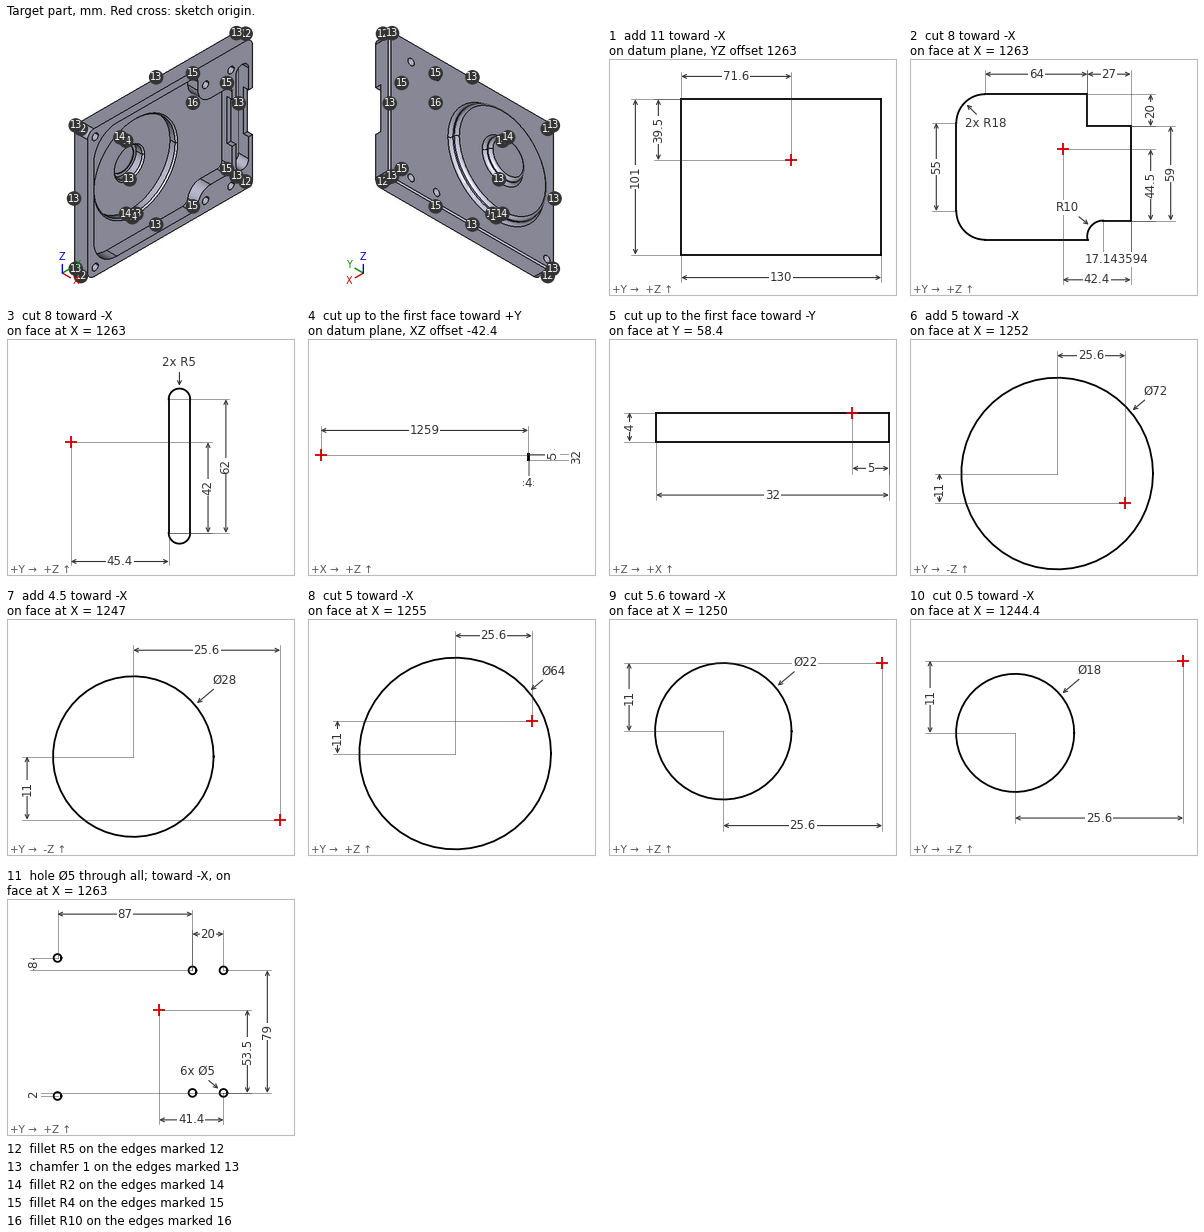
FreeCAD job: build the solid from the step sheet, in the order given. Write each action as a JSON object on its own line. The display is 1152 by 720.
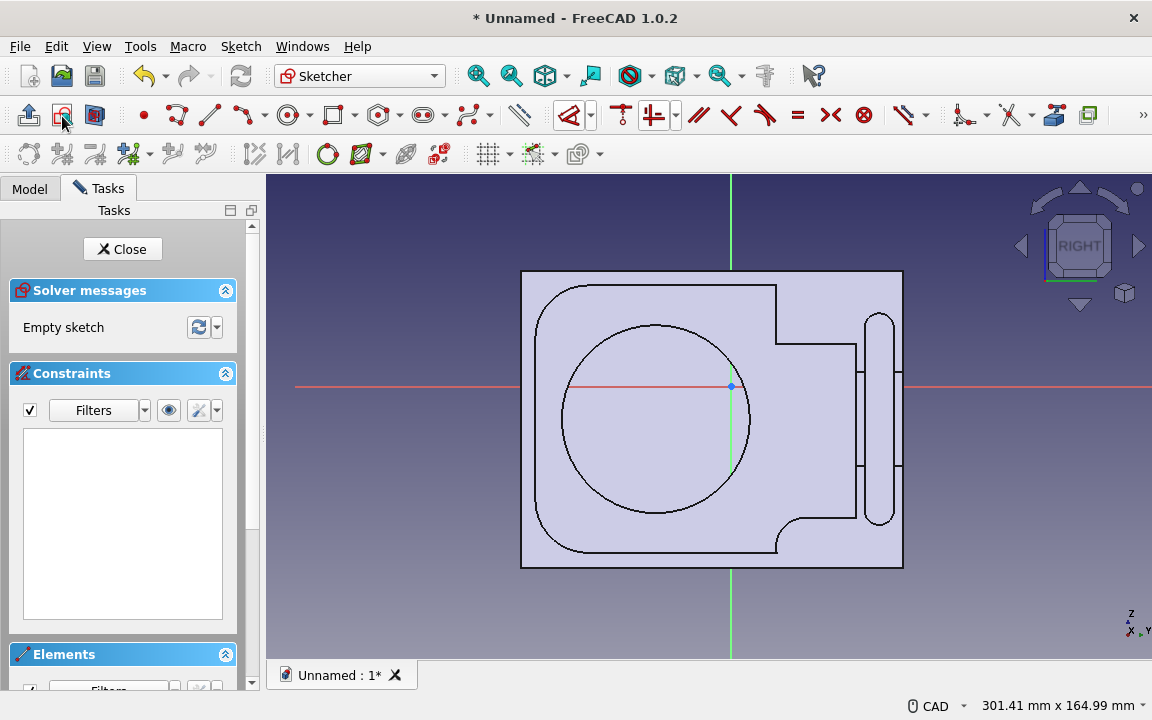
{"action": "left_click", "coordinate": [95, 116]}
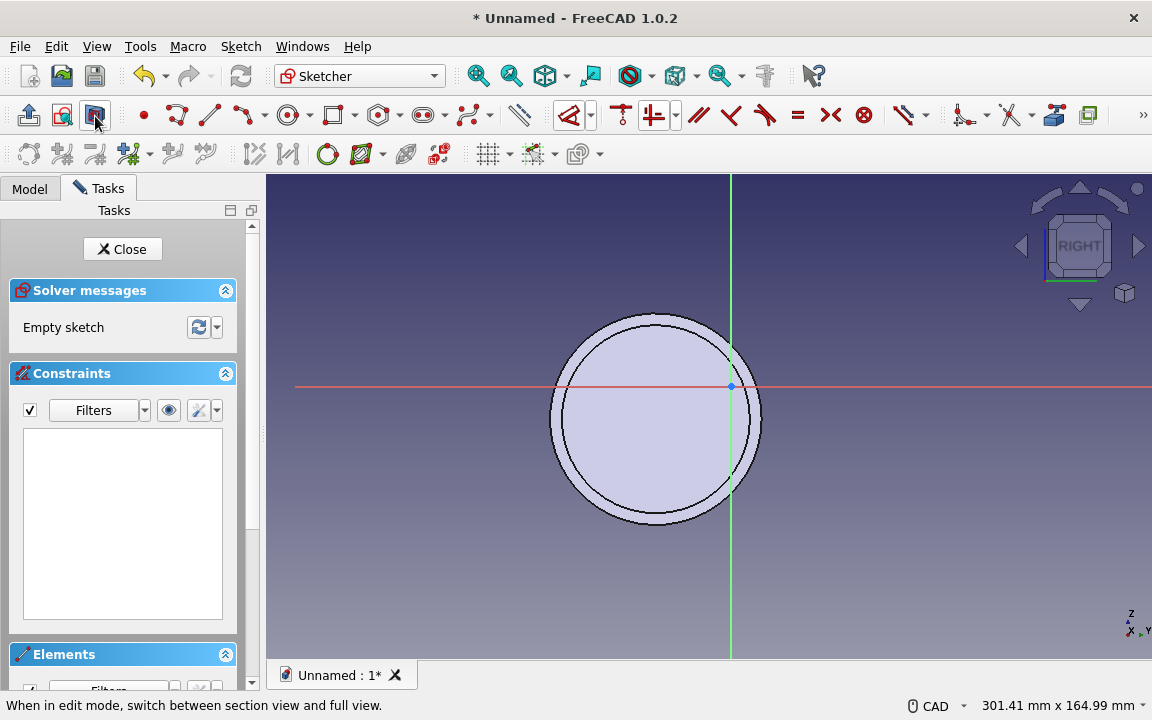
{"action": "scroll", "coordinate": [687, 420], "scroll_direction": "up", "scroll_amount": 8}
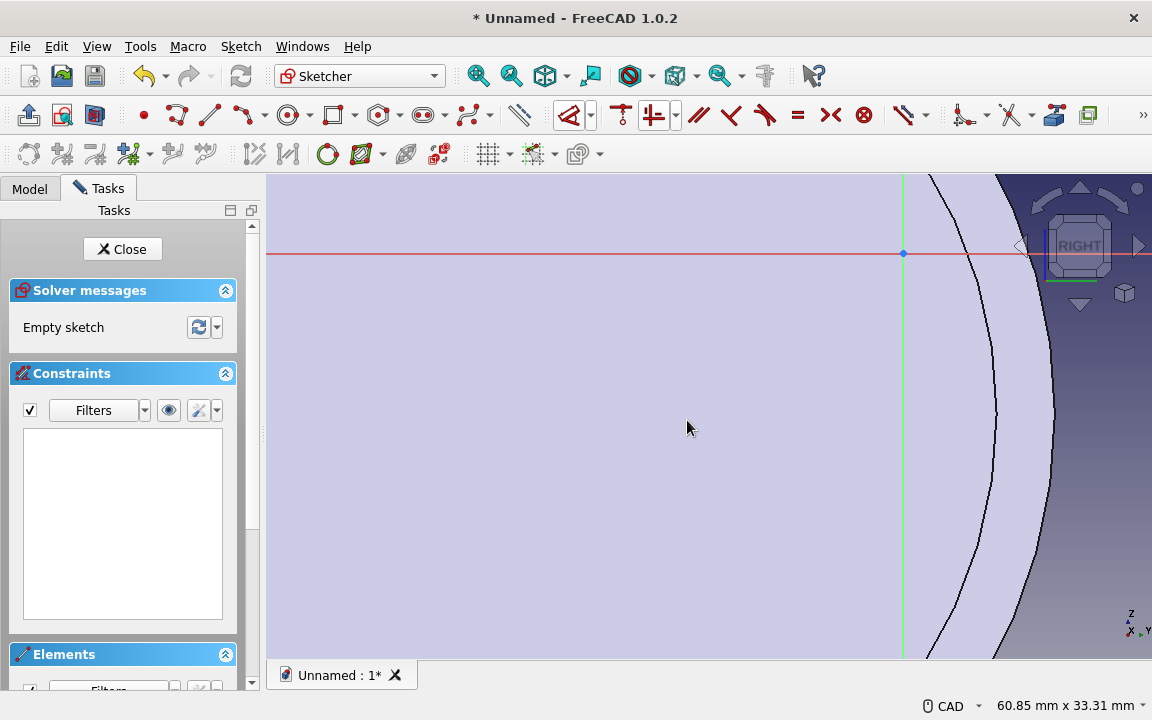
{"action": "left_click", "coordinate": [288, 116]}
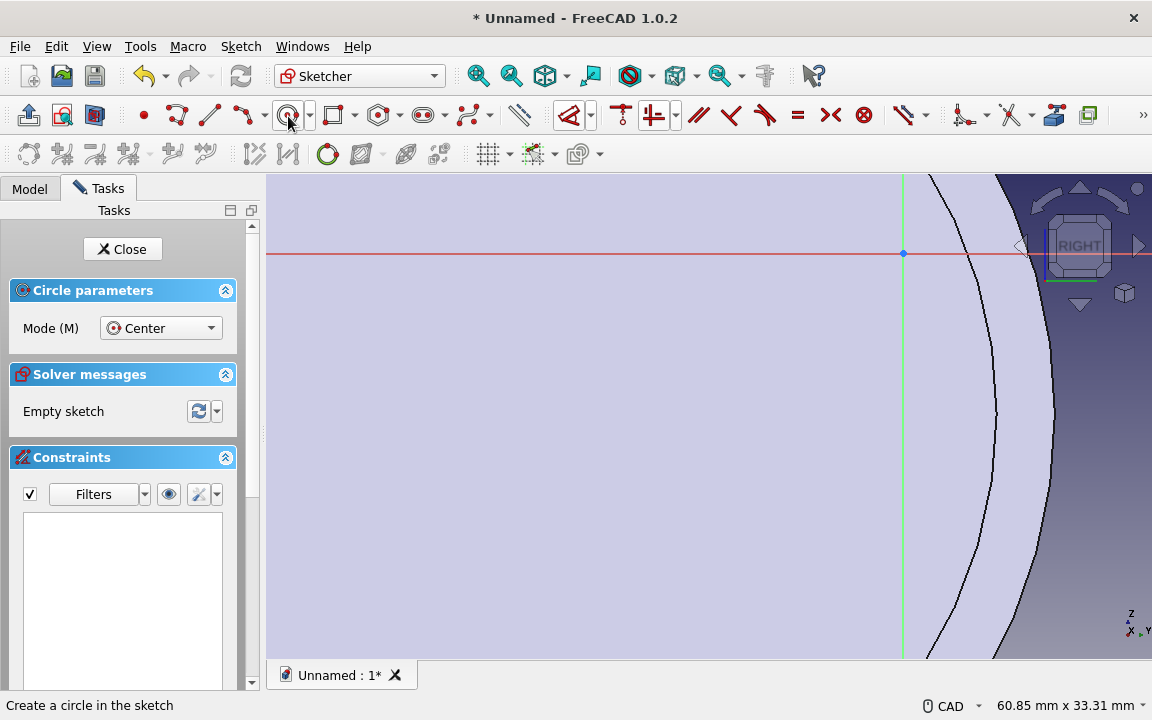
{"action": "left_click", "coordinate": [531, 414]}
{"action": "left_click", "coordinate": [644, 301]}
{"action": "key", "text": "Escape"}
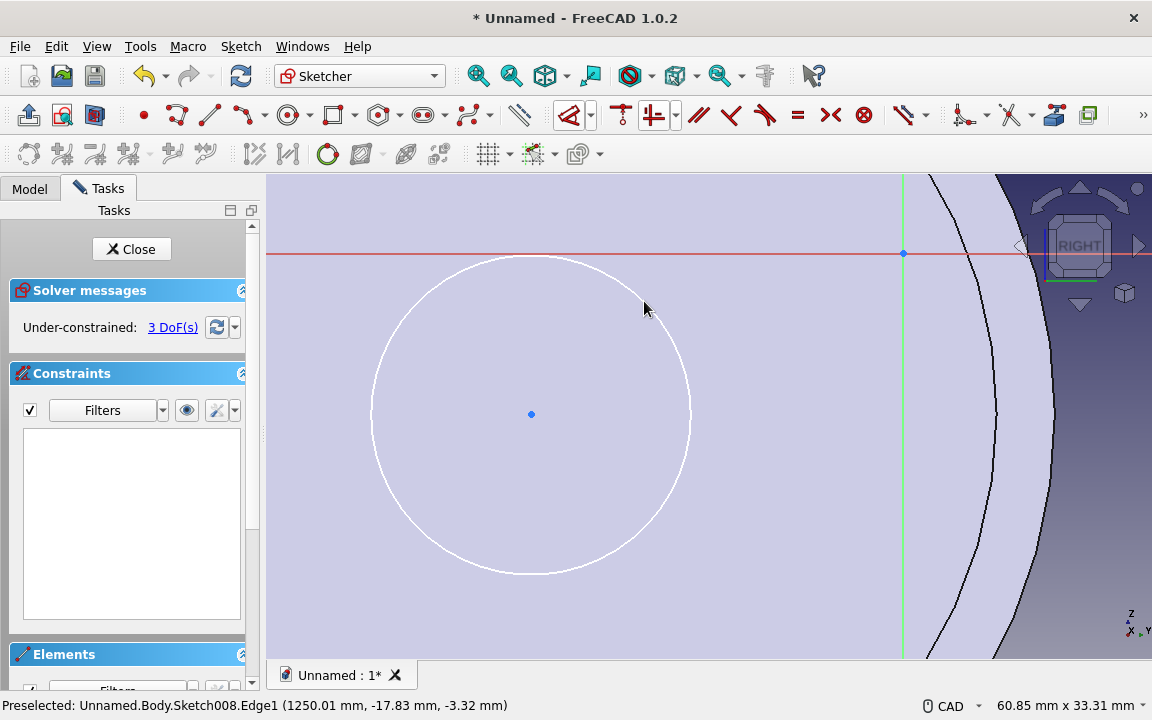
{"action": "left_click", "coordinate": [644, 302]}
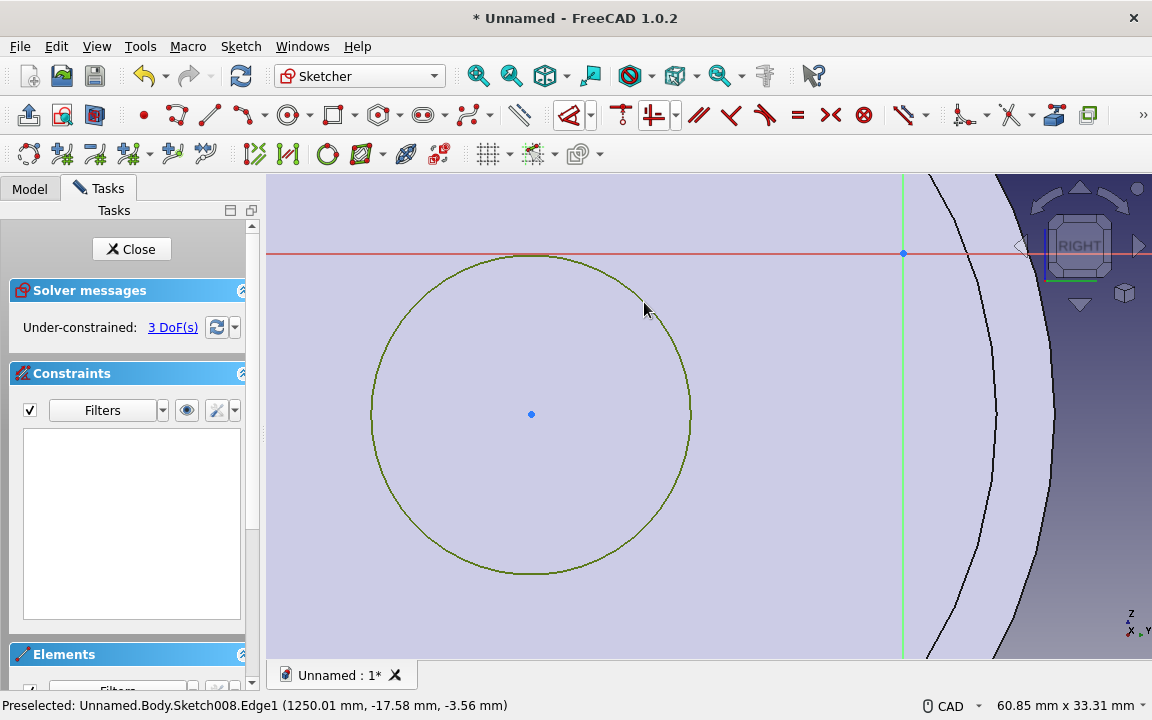
{"action": "key", "text": "k o"}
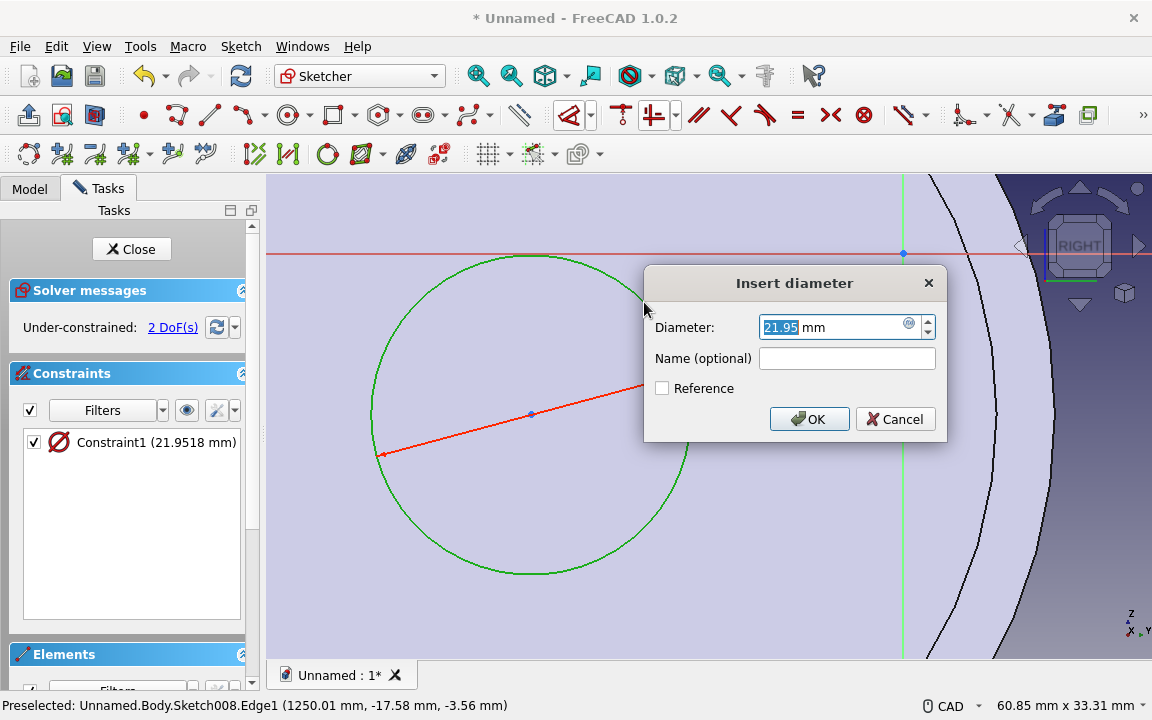
{"action": "type", "text": "22"}
{"action": "key", "text": "Return"}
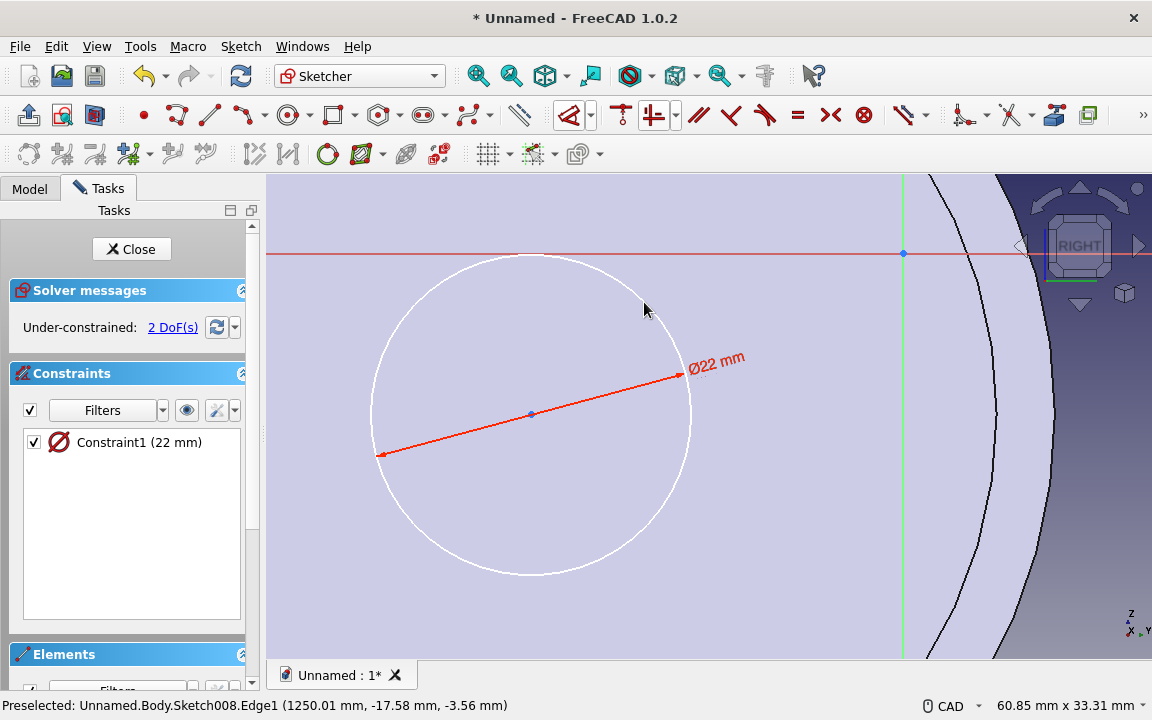
{"action": "left_click", "coordinate": [531, 415]}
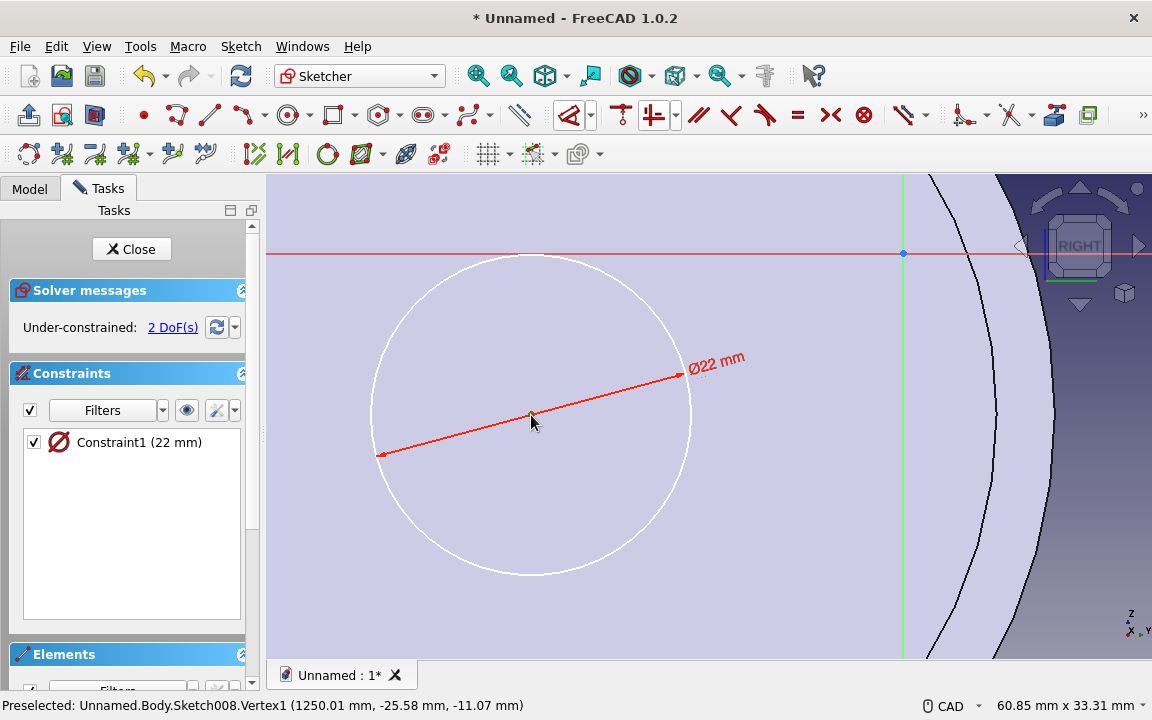
{"action": "key", "text": "i"}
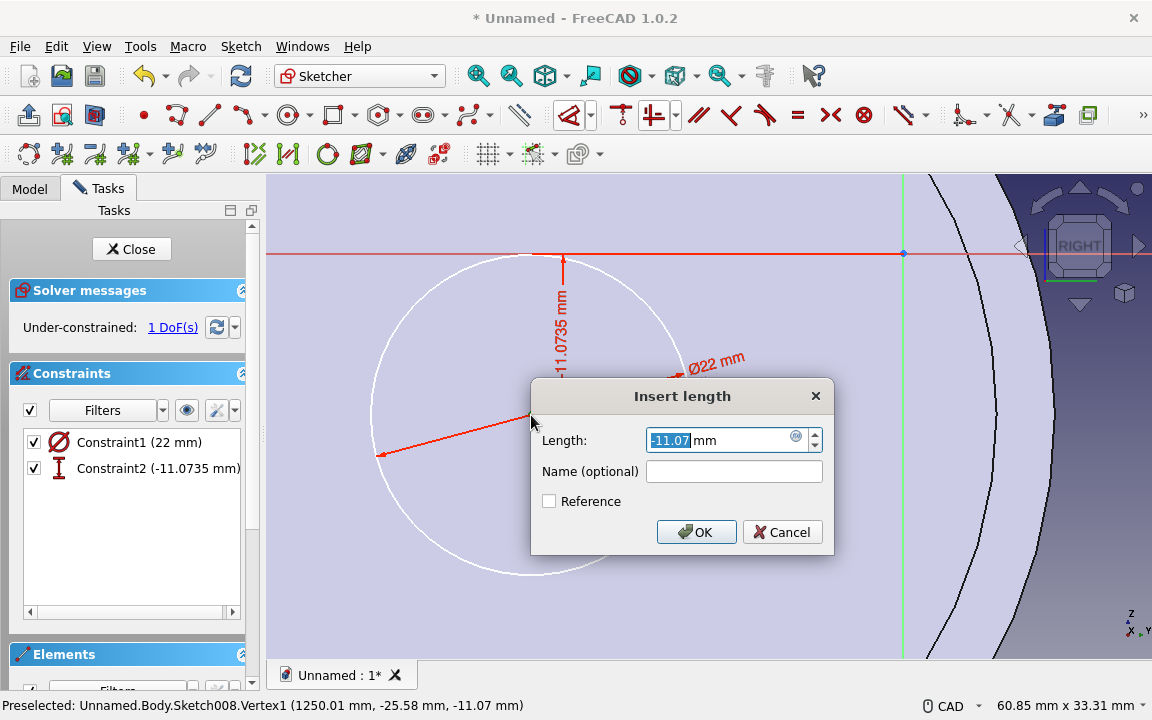
{"action": "type", "text": "-11"}
{"action": "key", "text": "Return"}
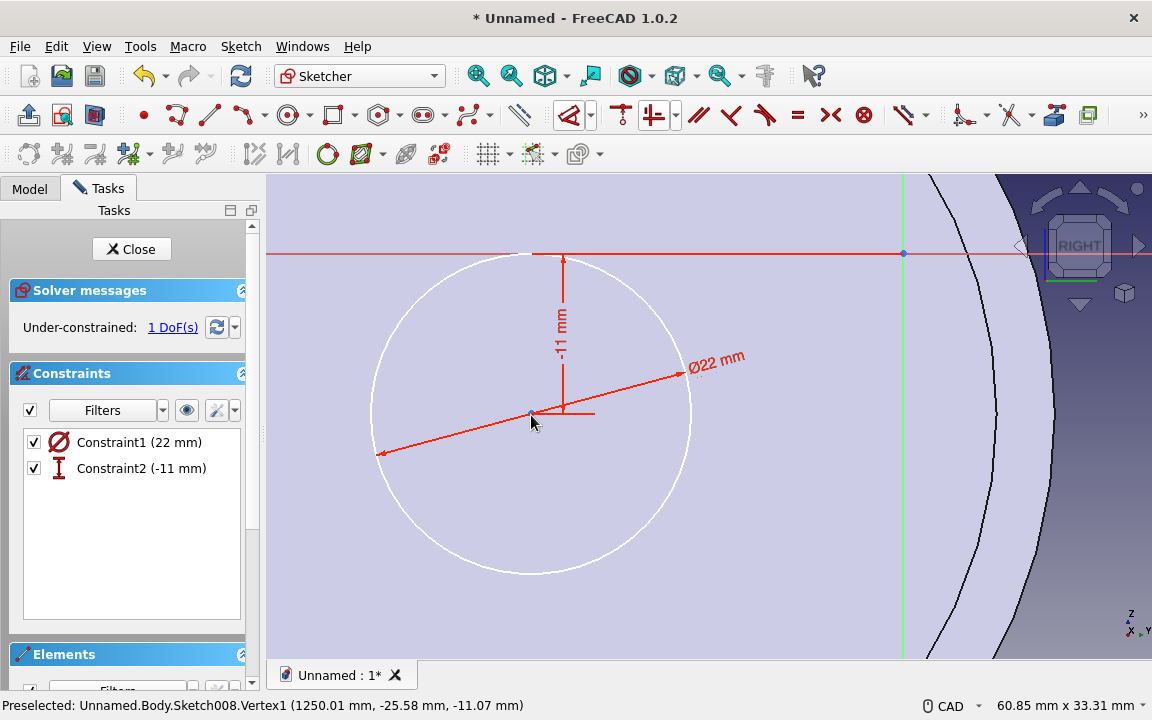
{"action": "left_click", "coordinate": [531, 414]}